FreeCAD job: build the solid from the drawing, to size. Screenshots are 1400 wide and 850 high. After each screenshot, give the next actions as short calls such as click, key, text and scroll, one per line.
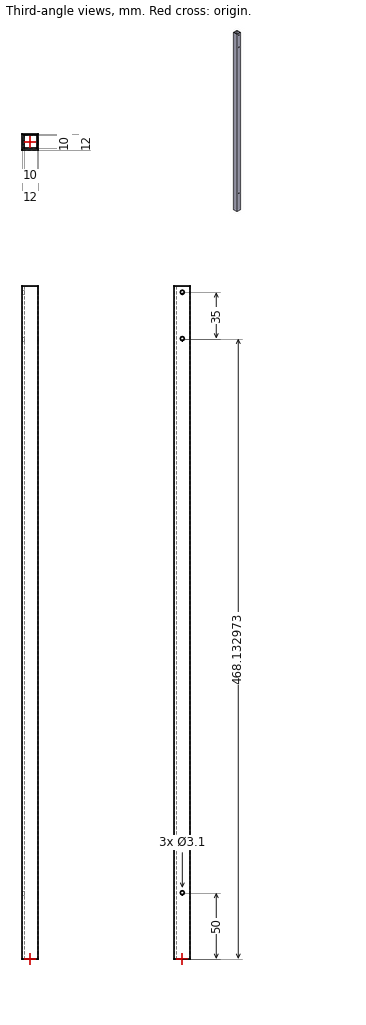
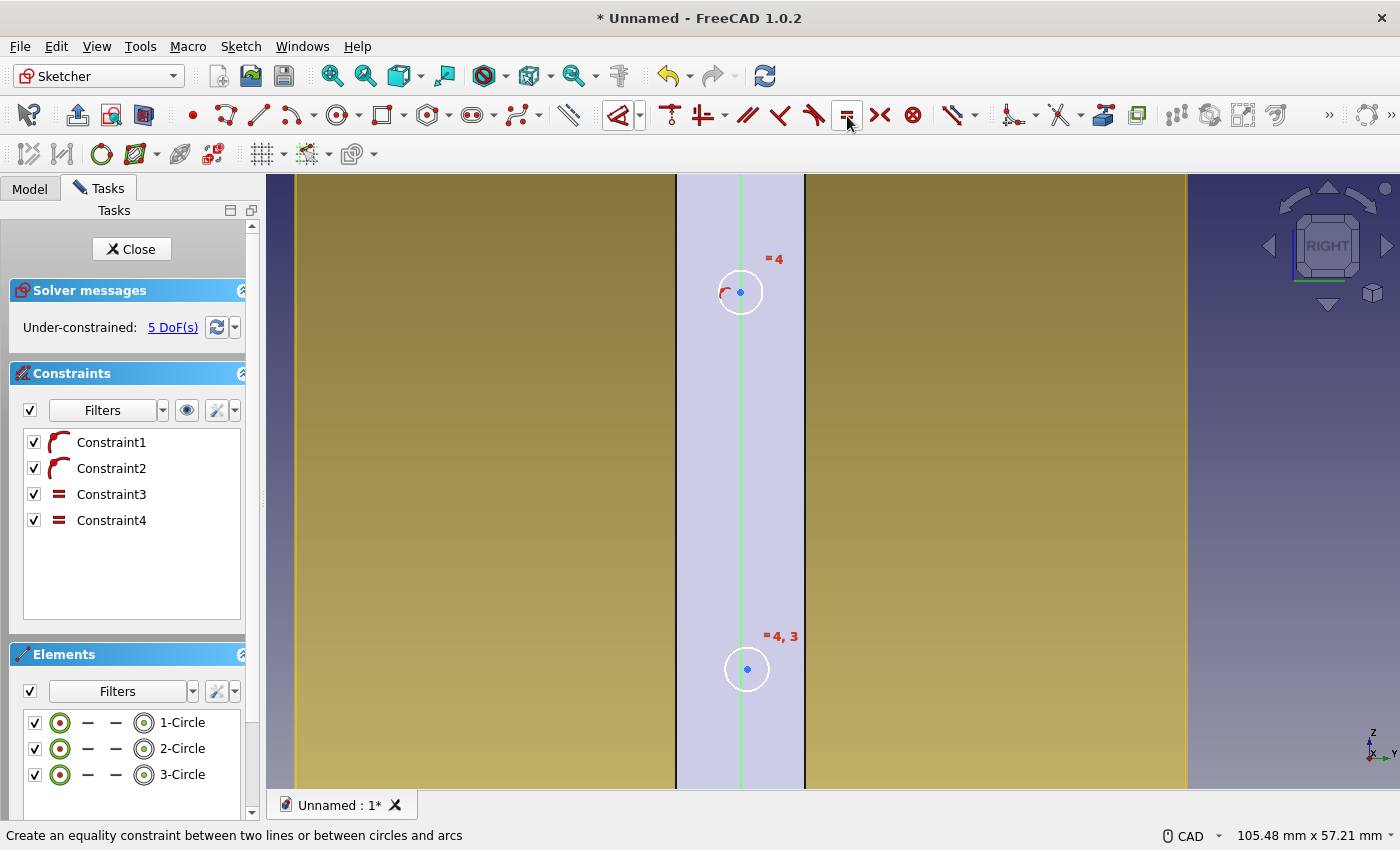
scroll(766, 281, down, 13)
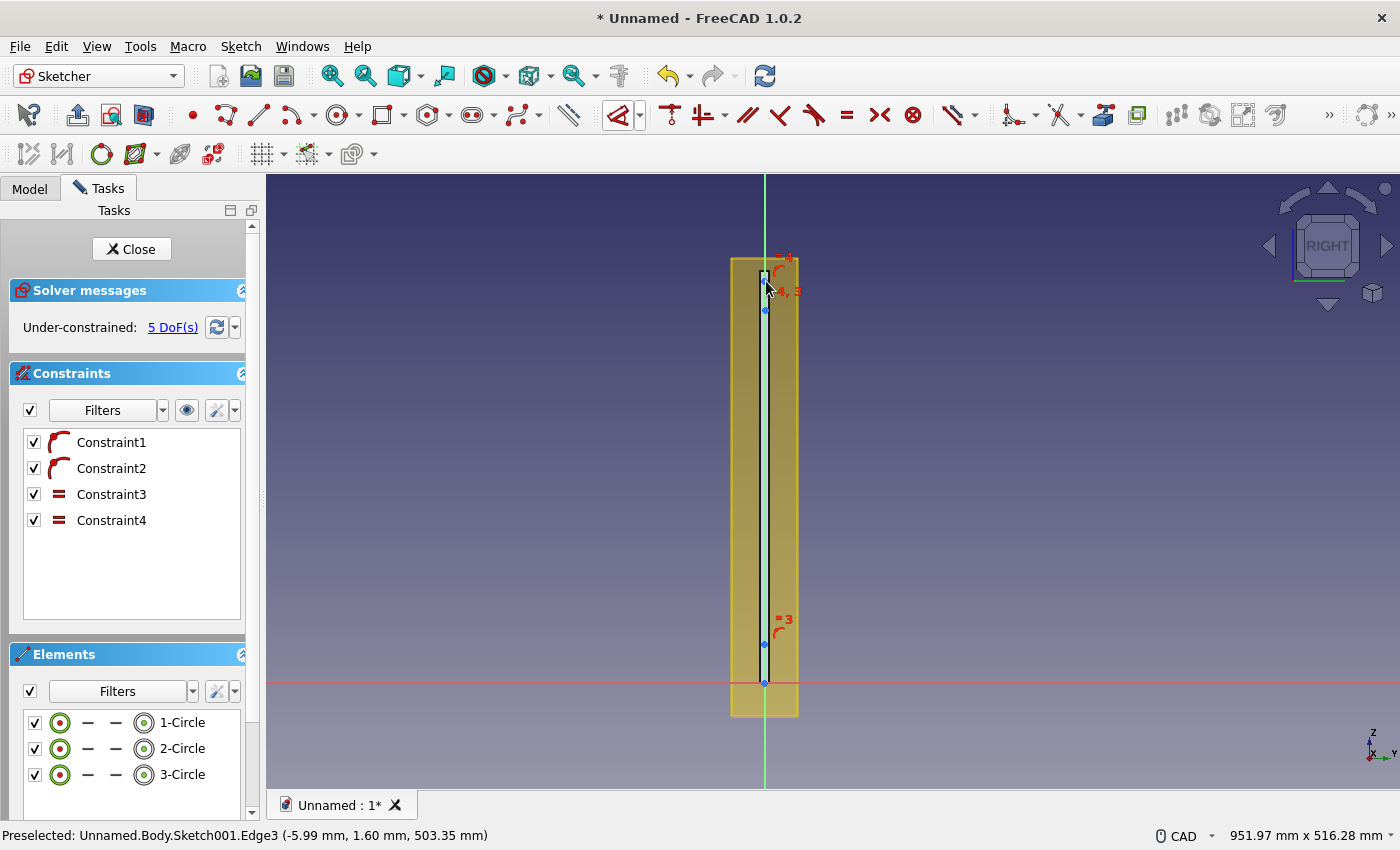
click(765, 310)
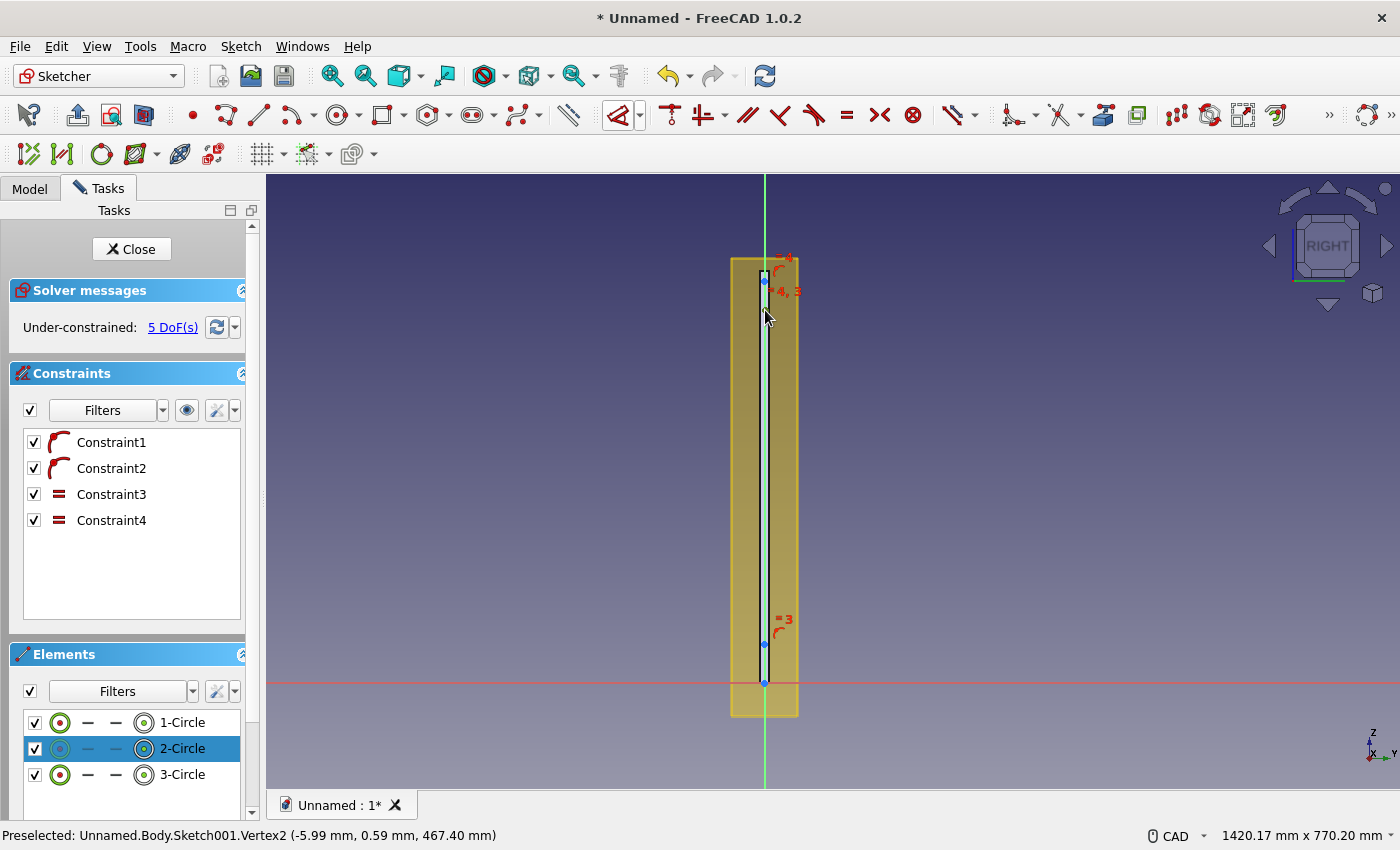
click(765, 721)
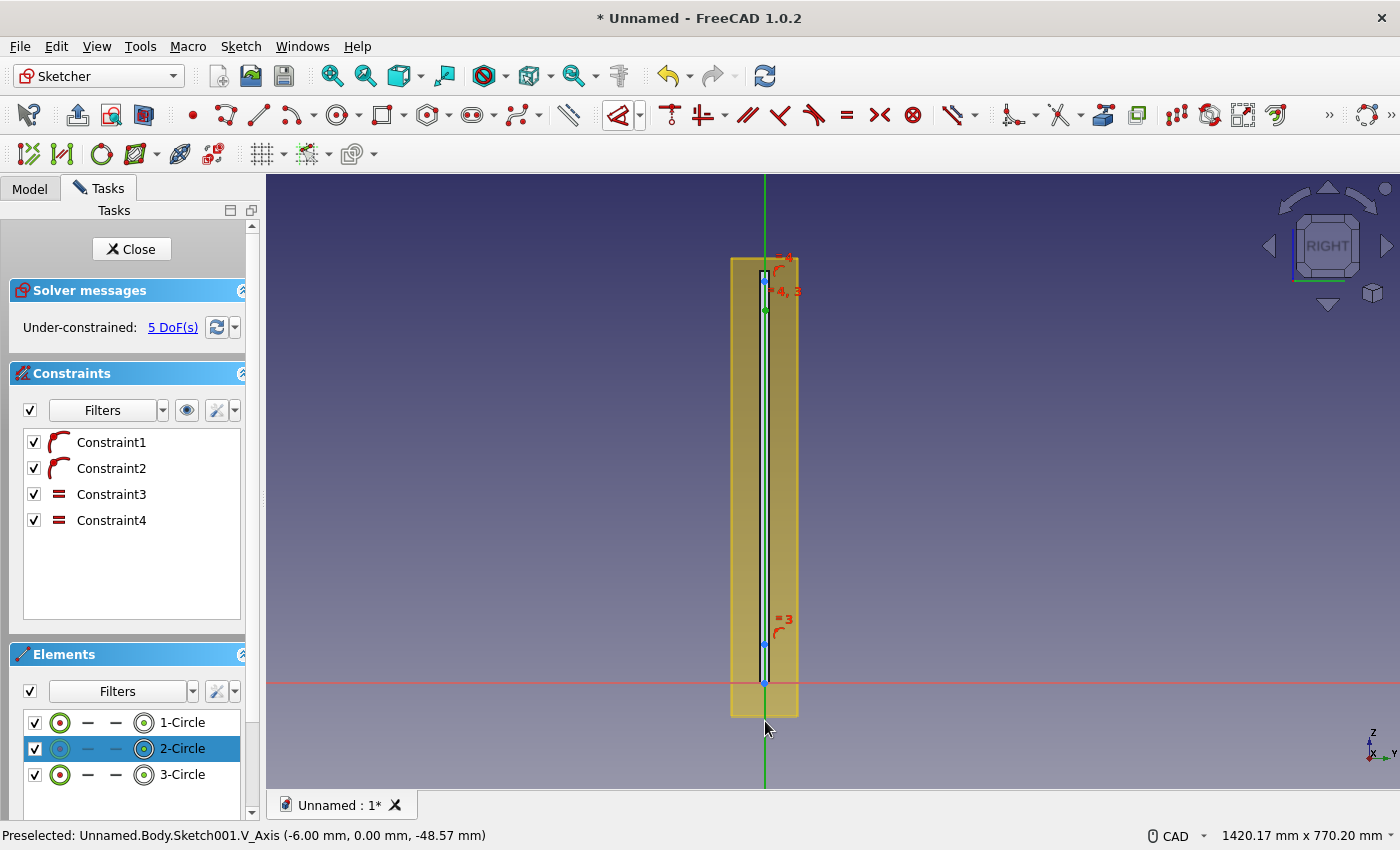
click(670, 116)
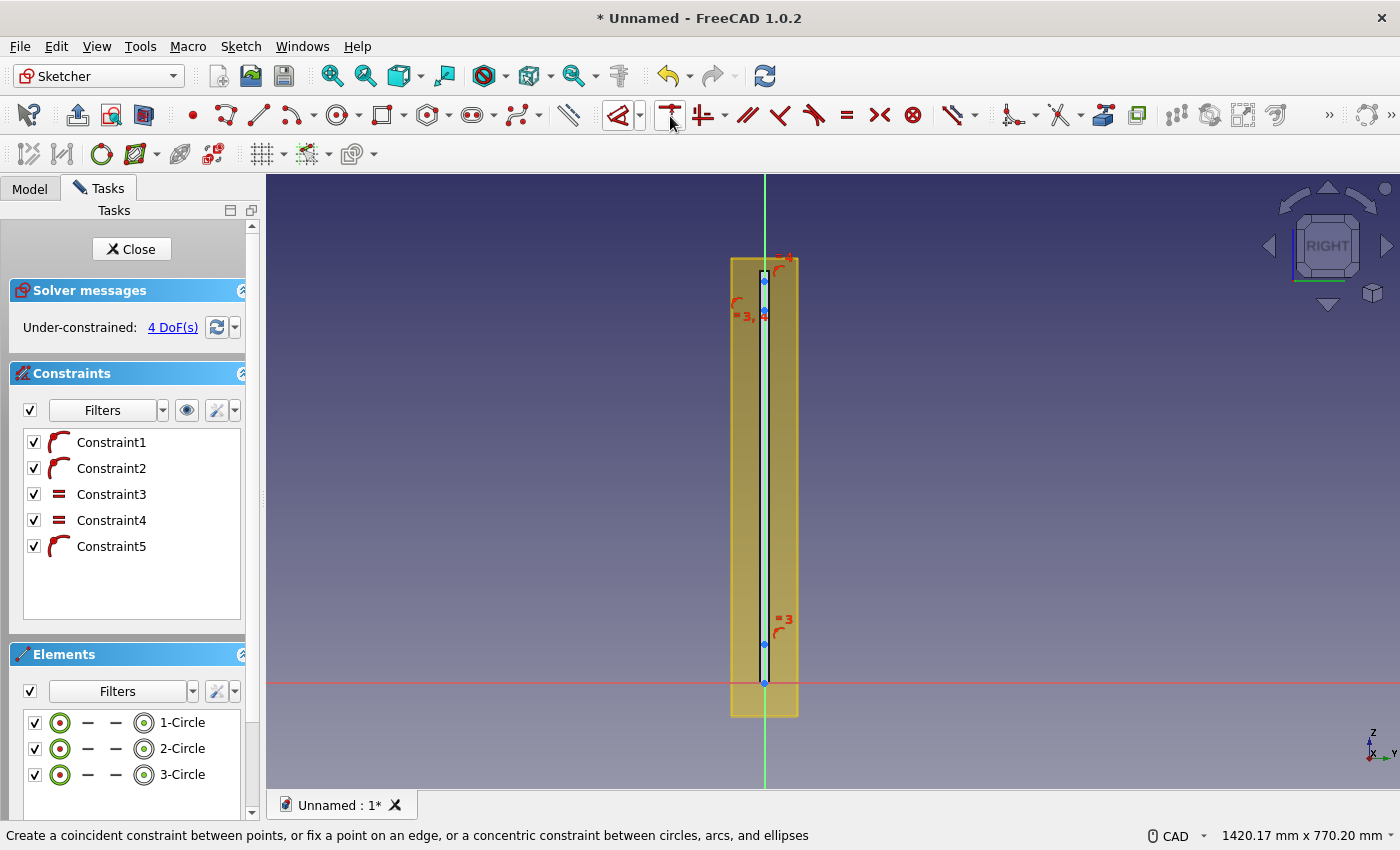
scroll(766, 645, up, 14)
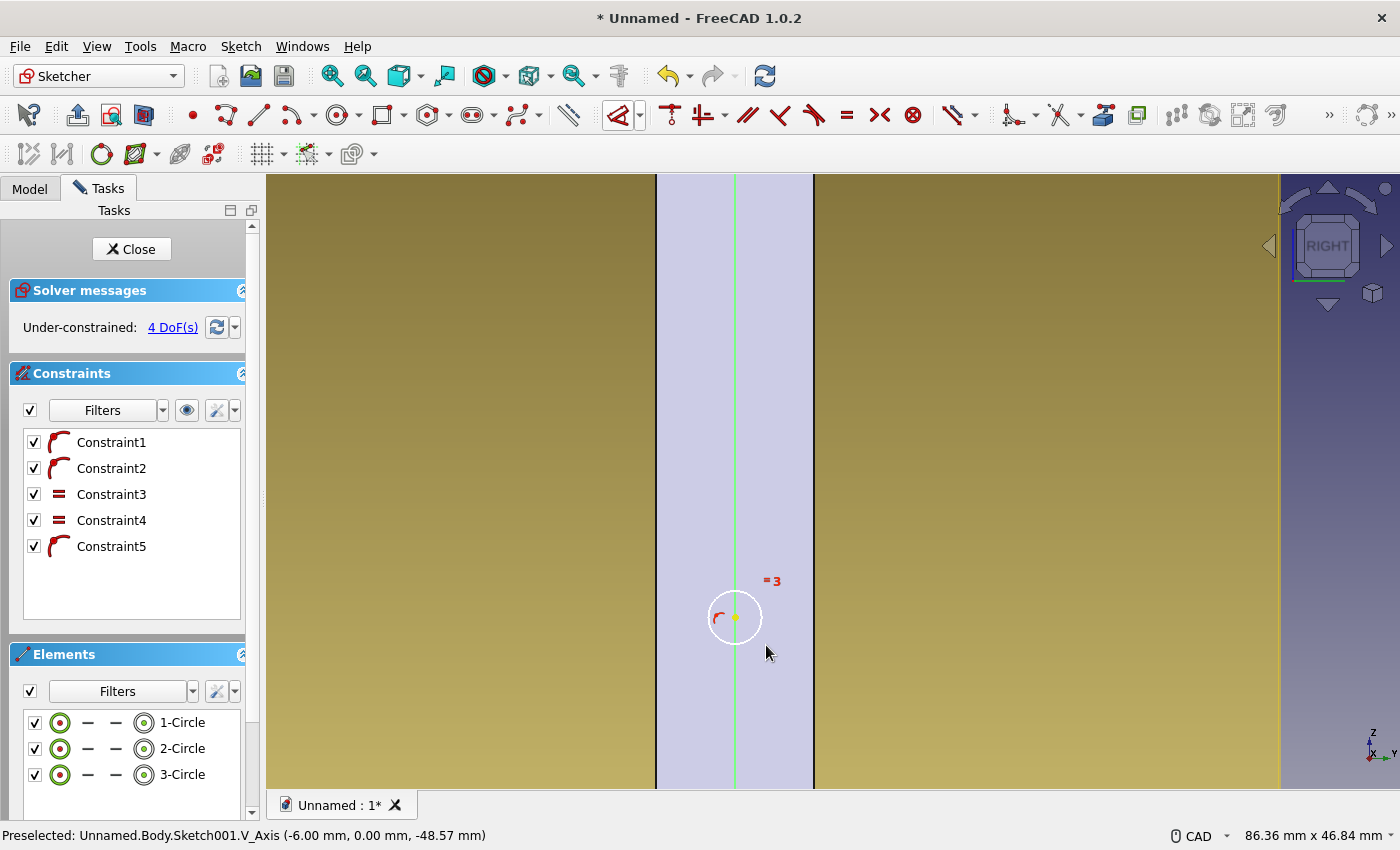
click(754, 636)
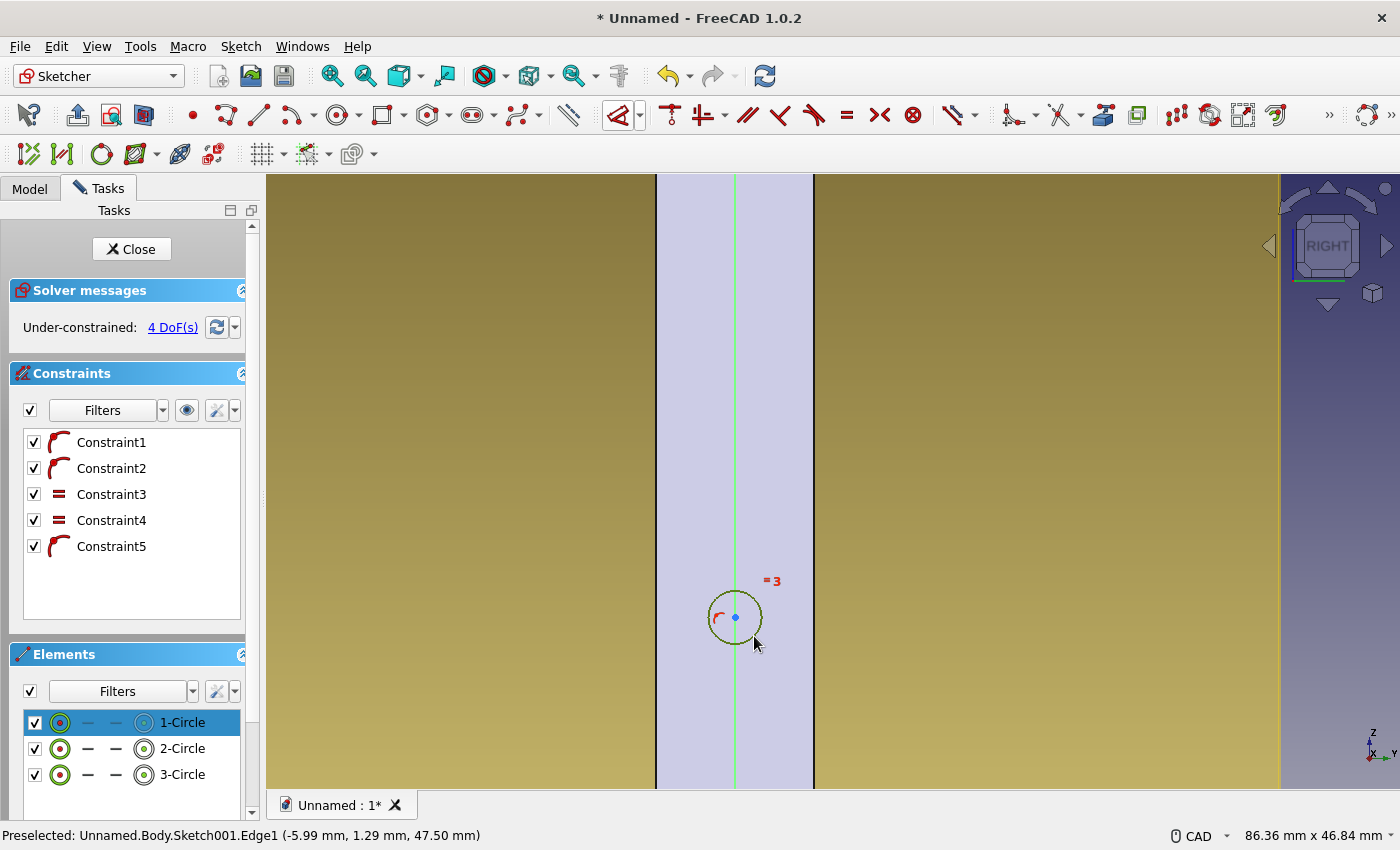
click(640, 116)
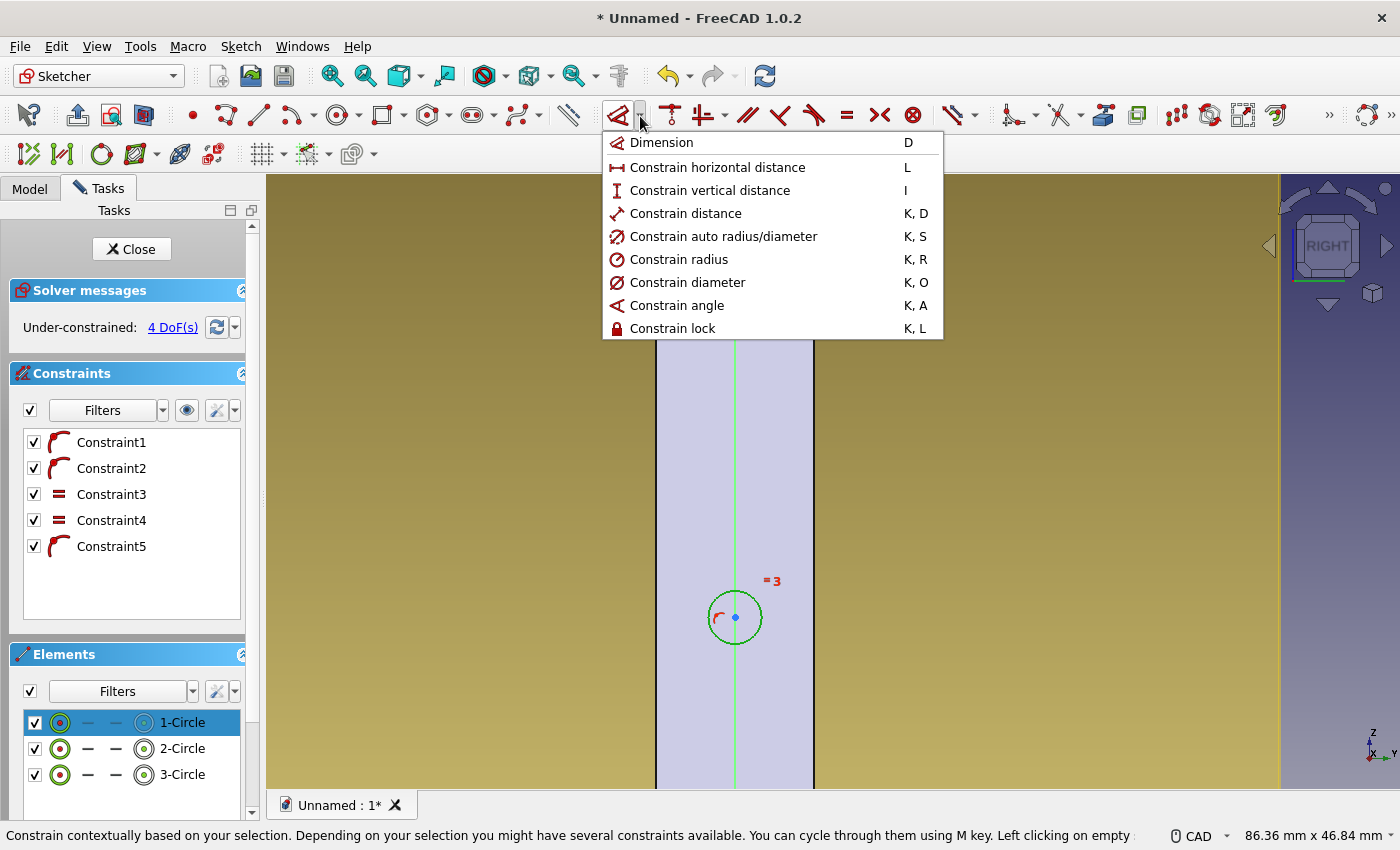
click(773, 282)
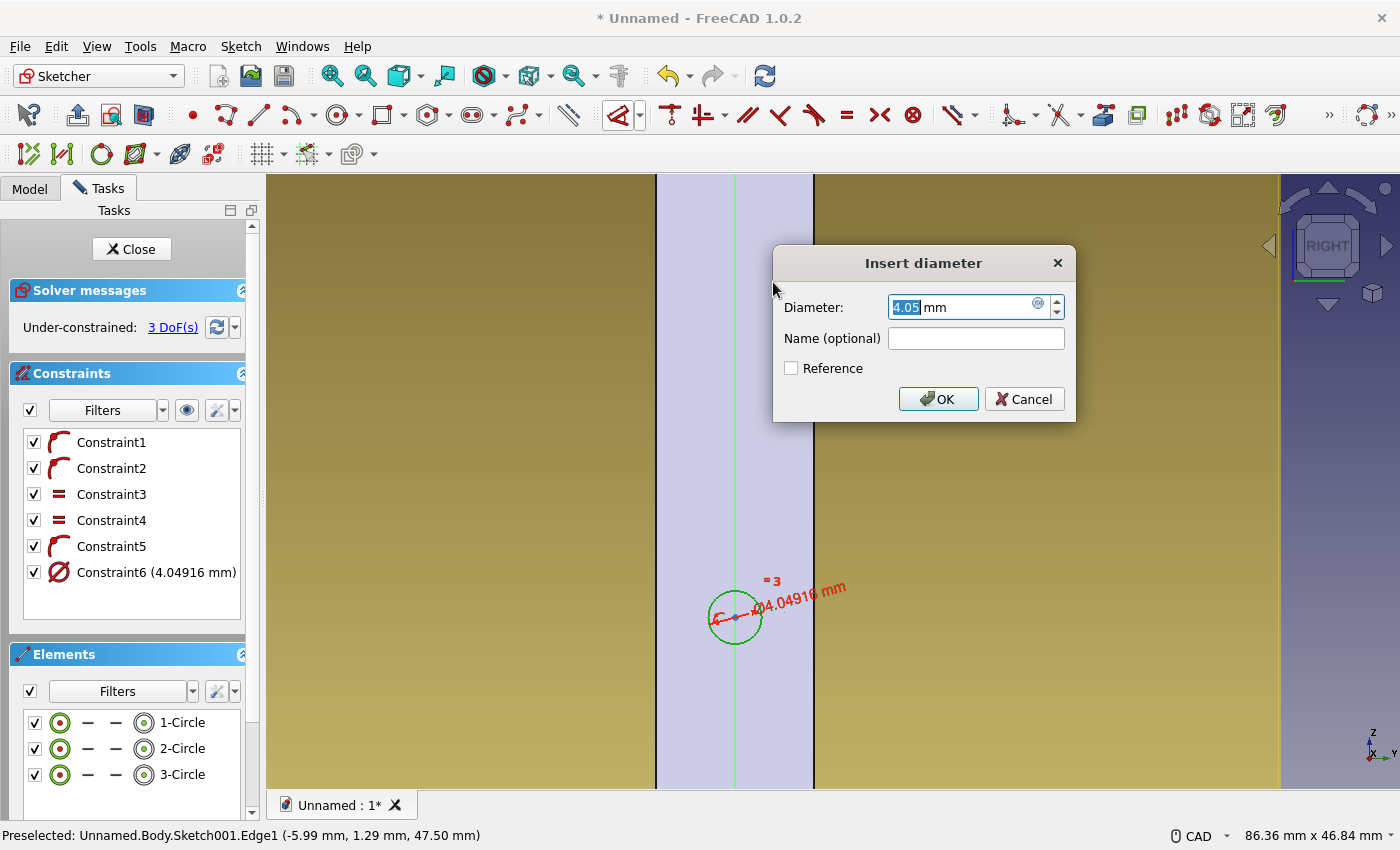
text(3.1)
key(Return)